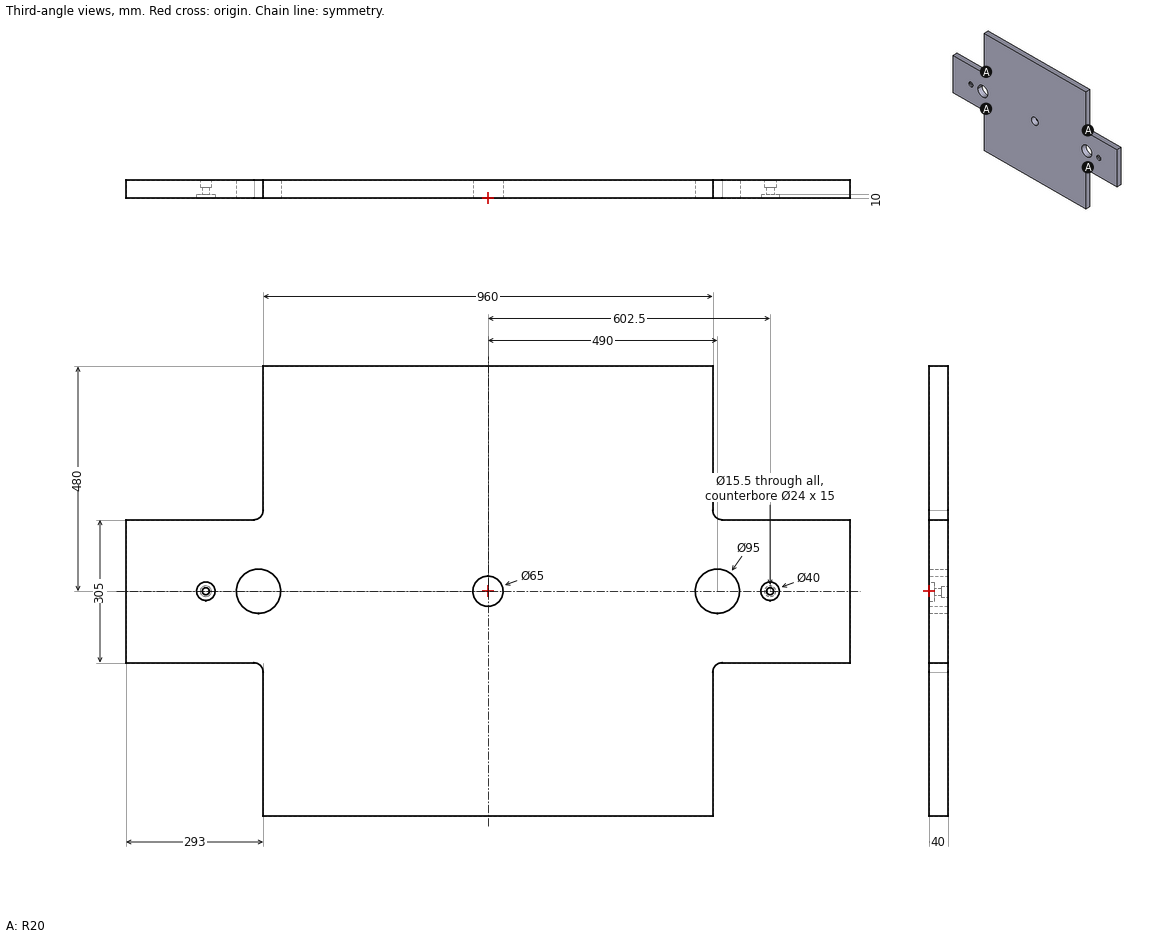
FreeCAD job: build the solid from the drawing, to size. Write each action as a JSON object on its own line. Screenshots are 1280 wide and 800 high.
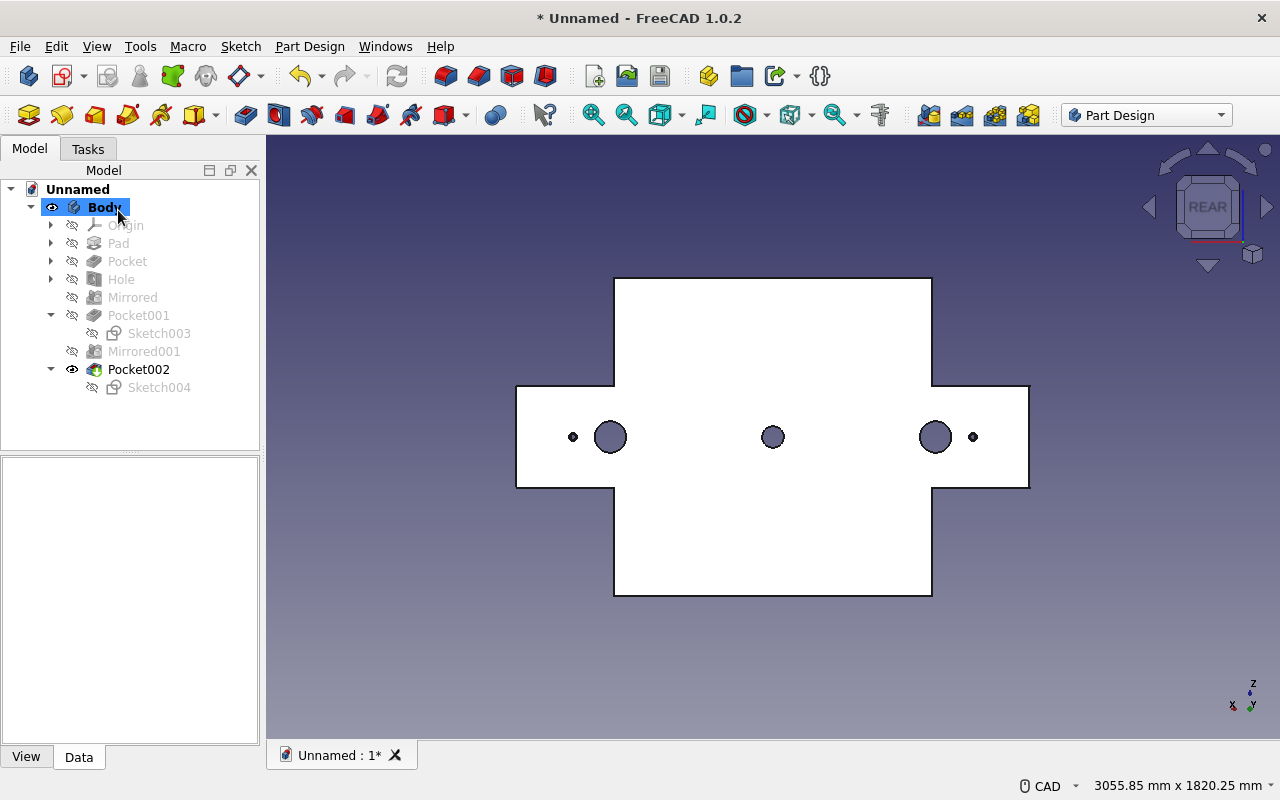
{"action": "scroll", "coordinate": [932, 385], "scroll_direction": "up", "scroll_amount": 6}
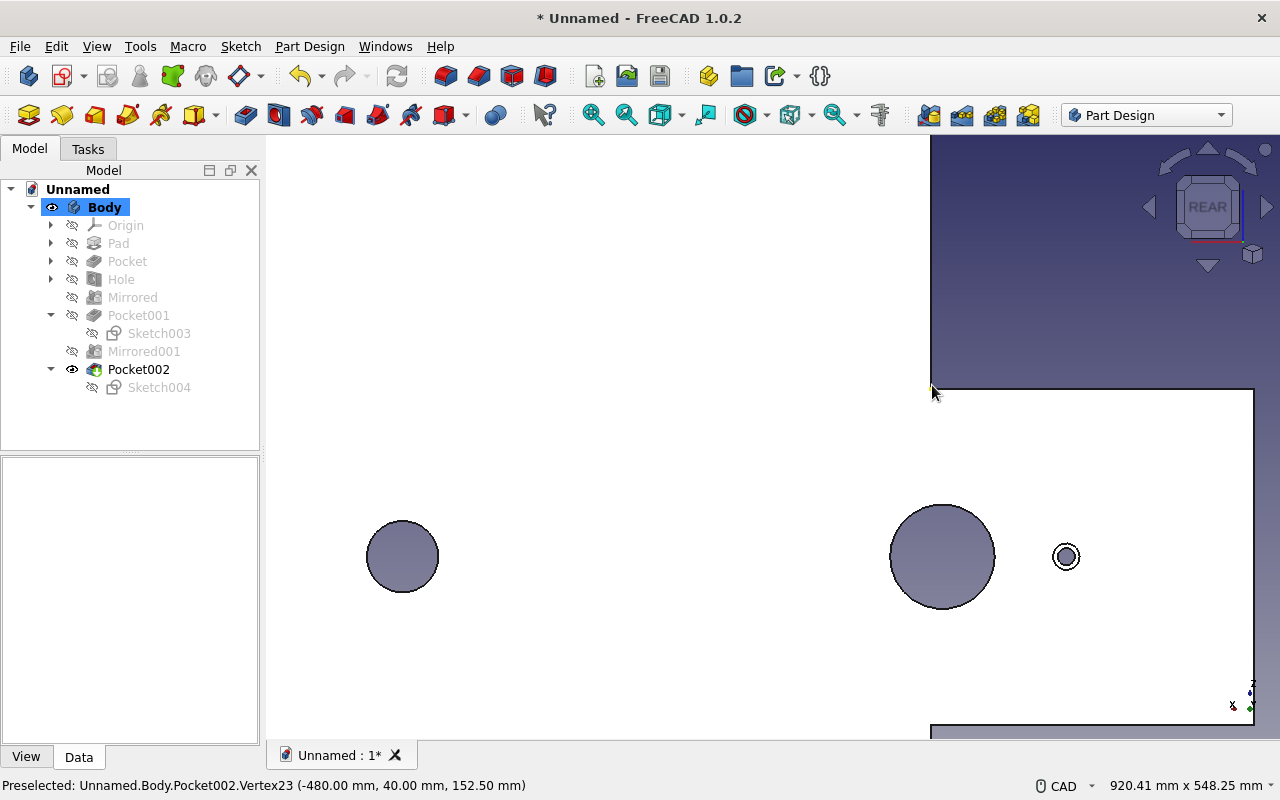
{"action": "left_click", "coordinate": [594, 116]}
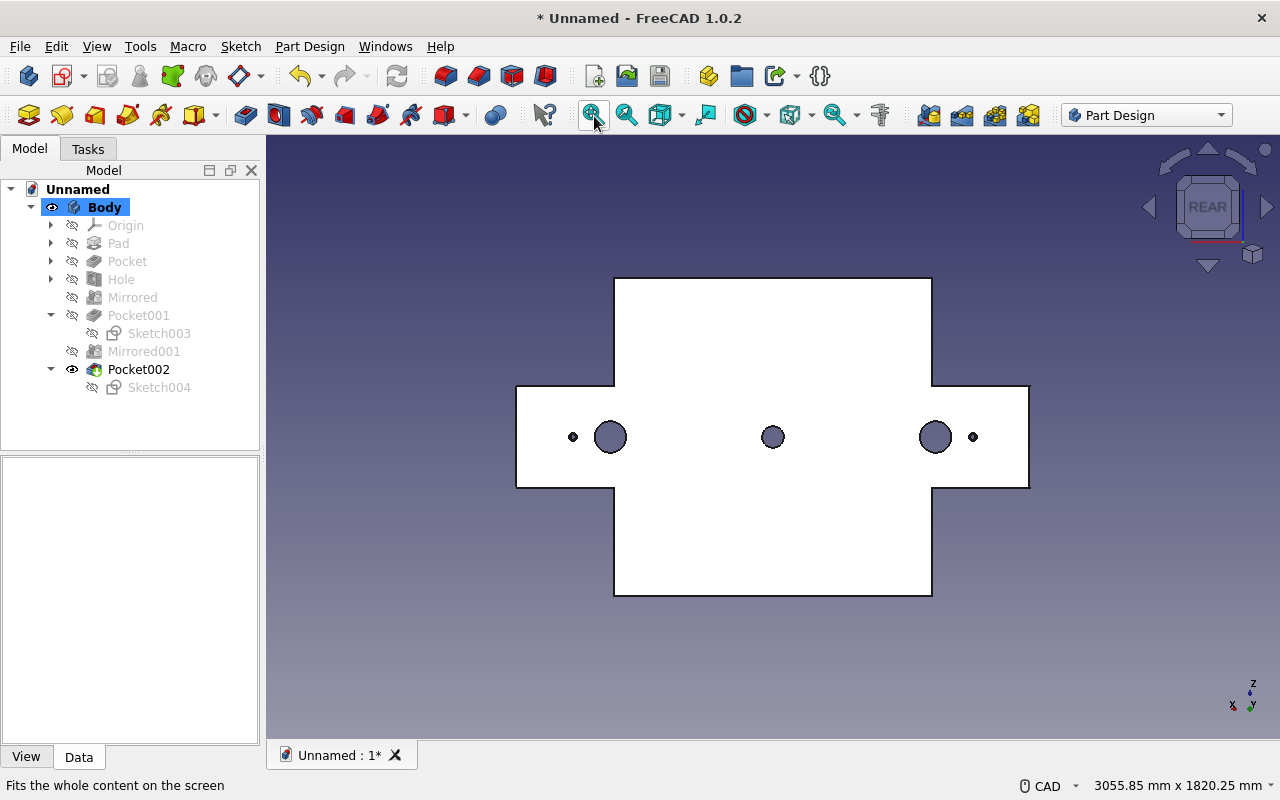
{"action": "key", "text": "0"}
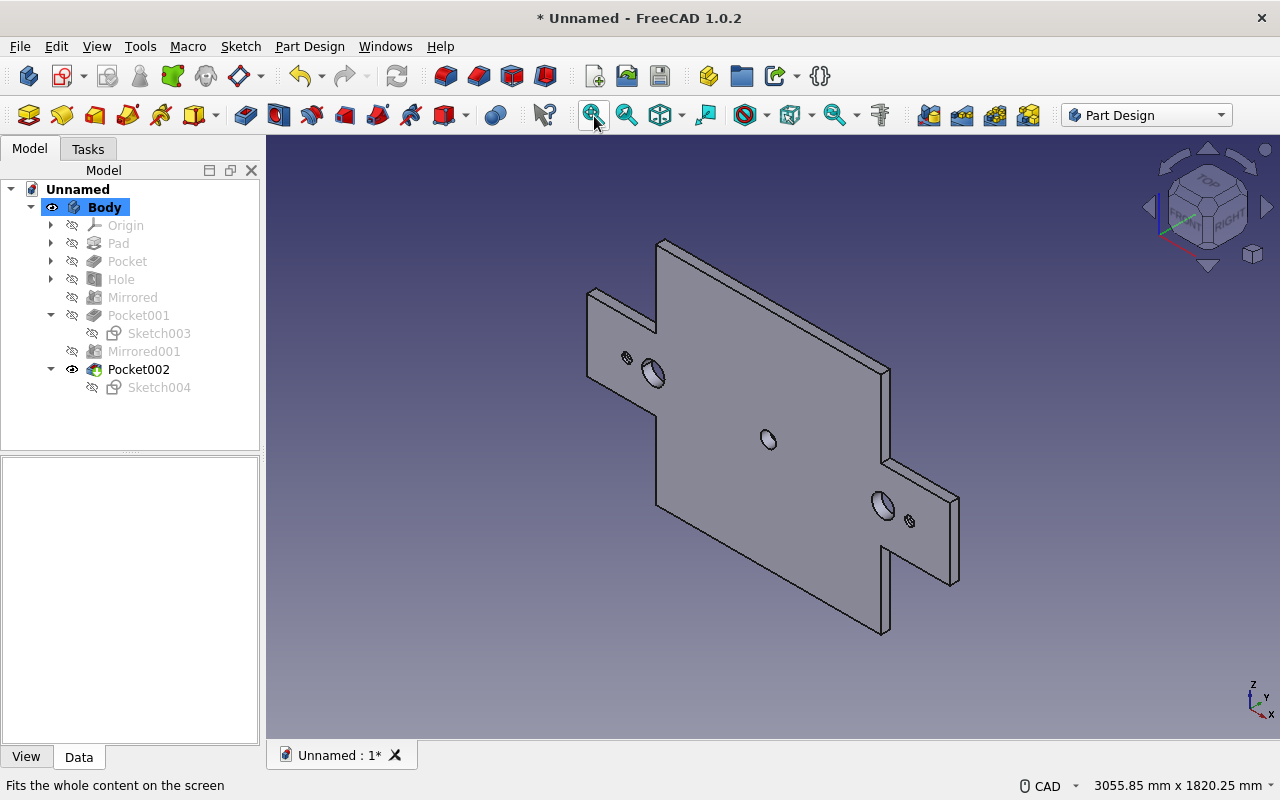
{"action": "scroll", "coordinate": [660, 330], "scroll_direction": "up", "scroll_amount": 6}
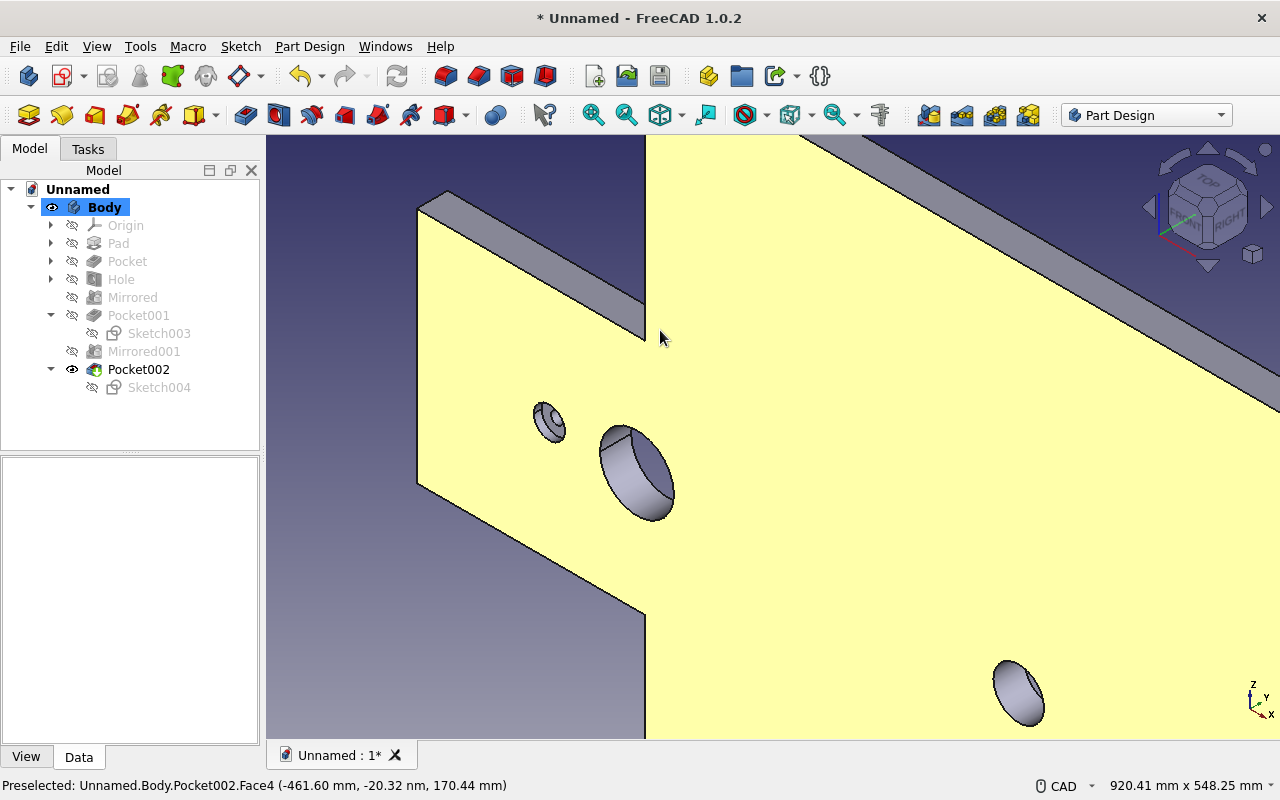
{"action": "key", "text": "v f"}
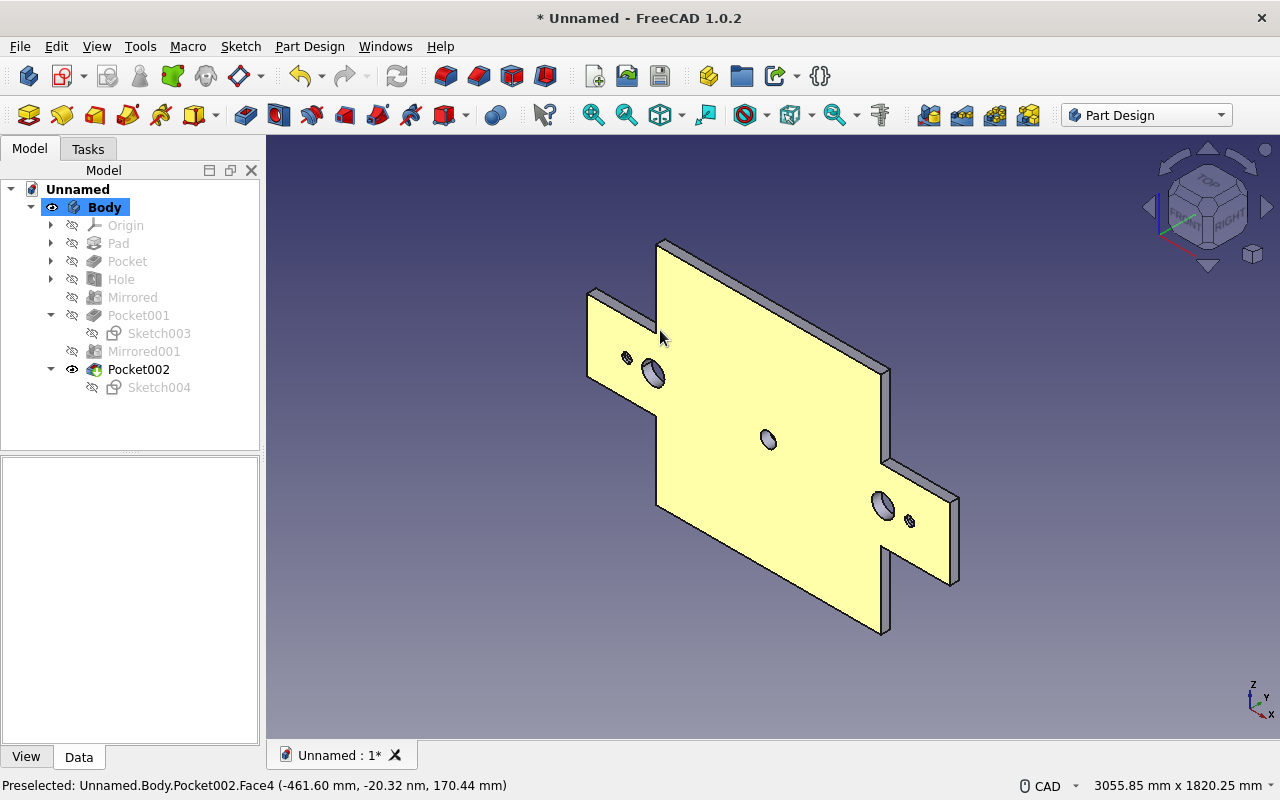
{"action": "key", "text": "2"}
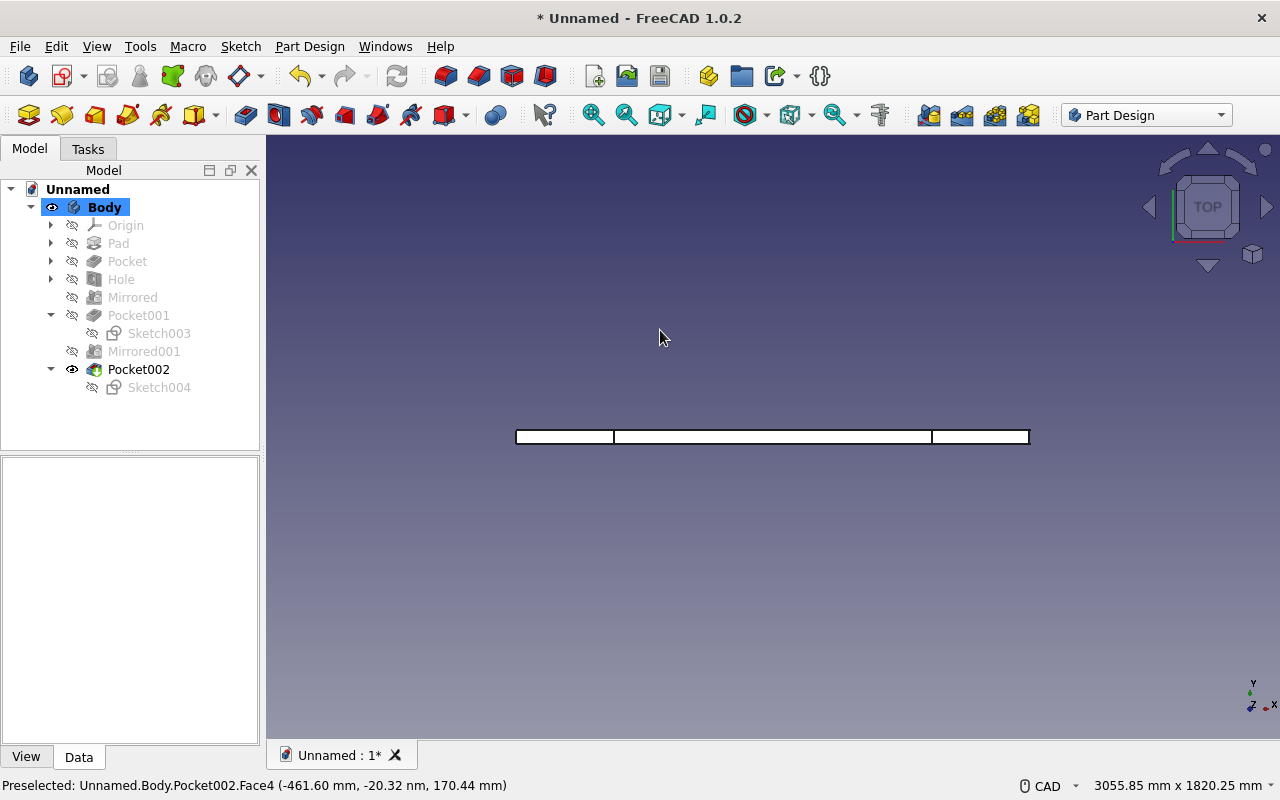
{"action": "scroll", "coordinate": [614, 436], "scroll_direction": "up", "scroll_amount": 6}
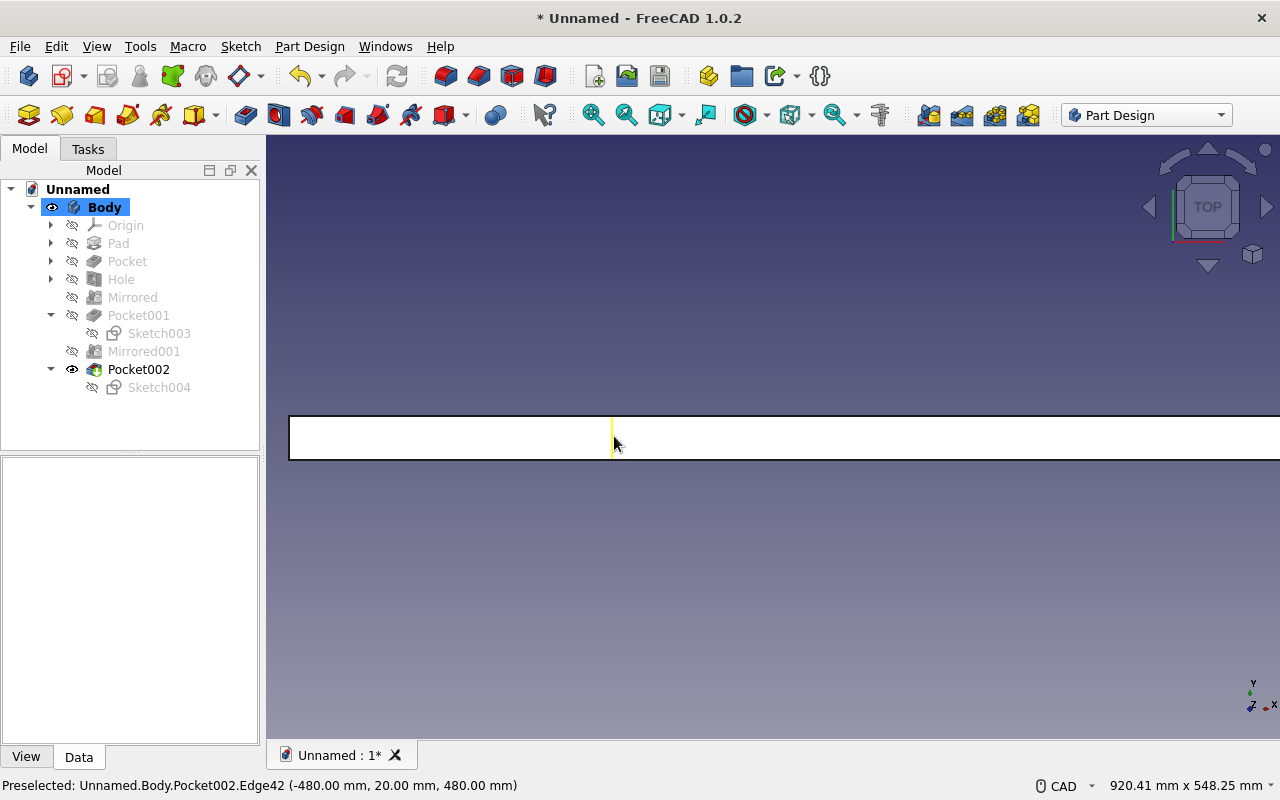
{"action": "key", "text": "v f"}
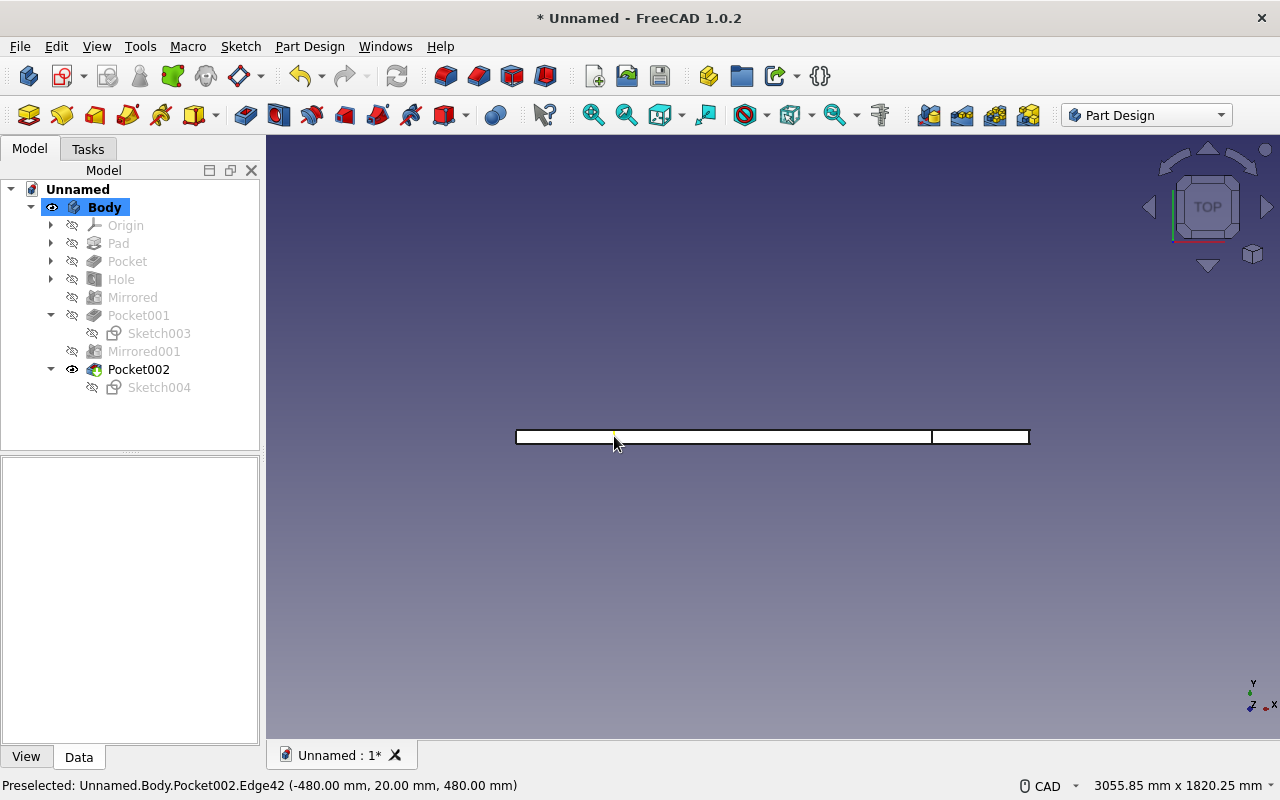
{"action": "key", "text": "1"}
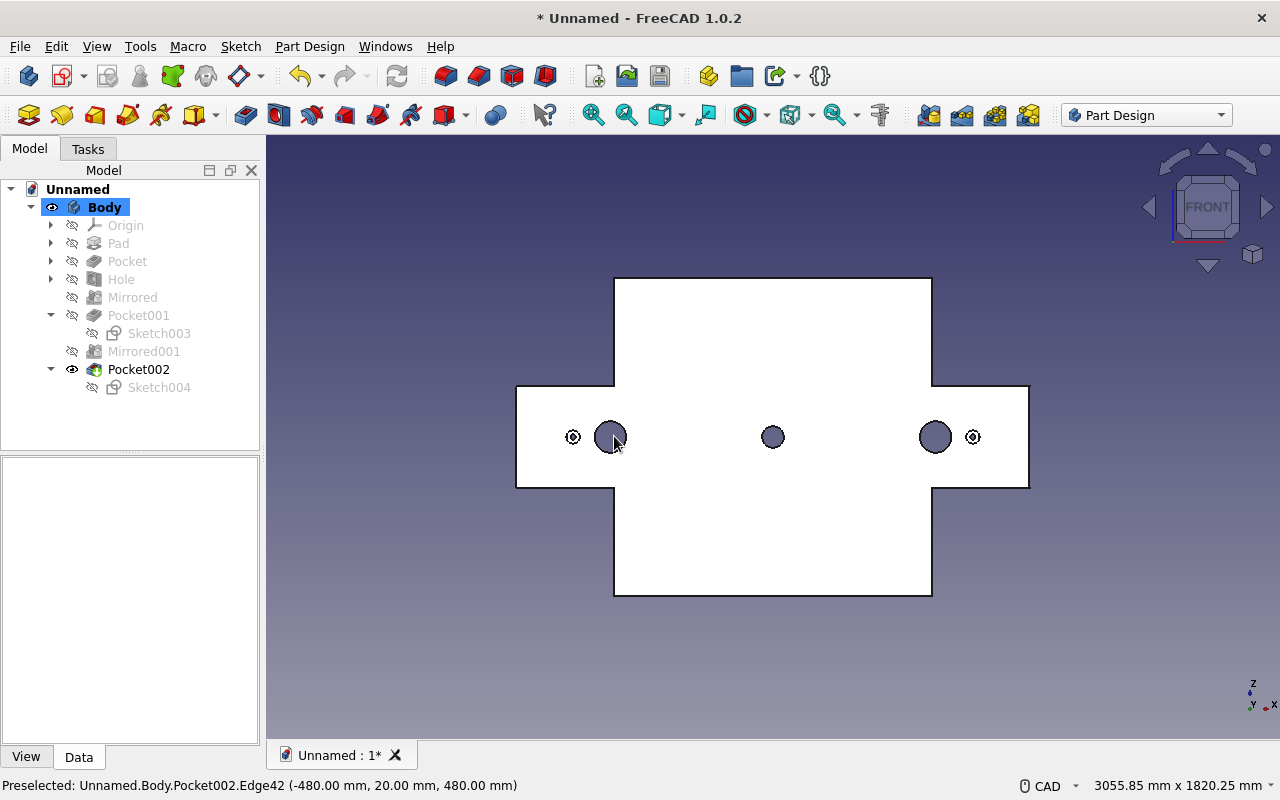
{"action": "scroll", "coordinate": [614, 385], "scroll_direction": "up", "scroll_amount": 6}